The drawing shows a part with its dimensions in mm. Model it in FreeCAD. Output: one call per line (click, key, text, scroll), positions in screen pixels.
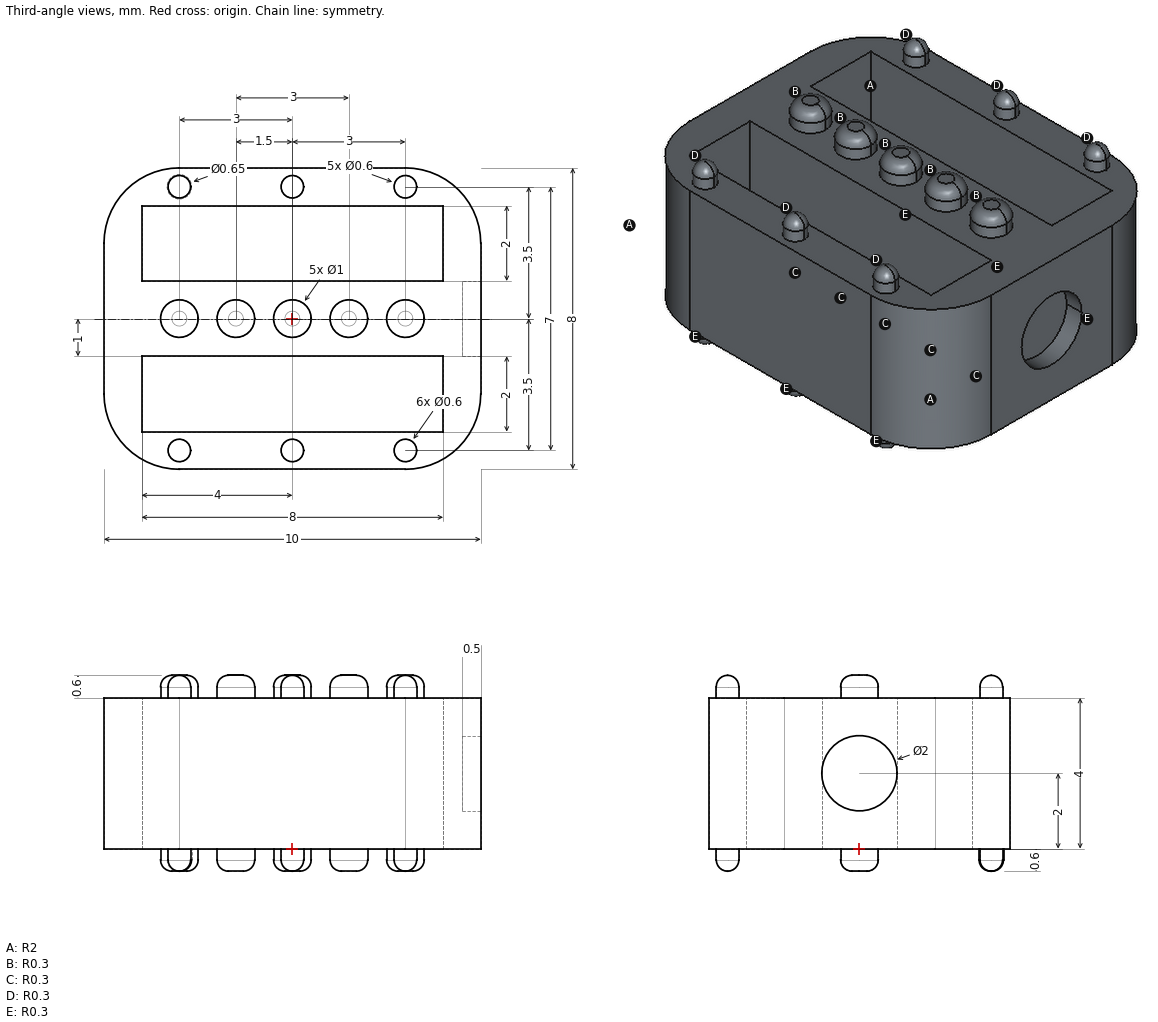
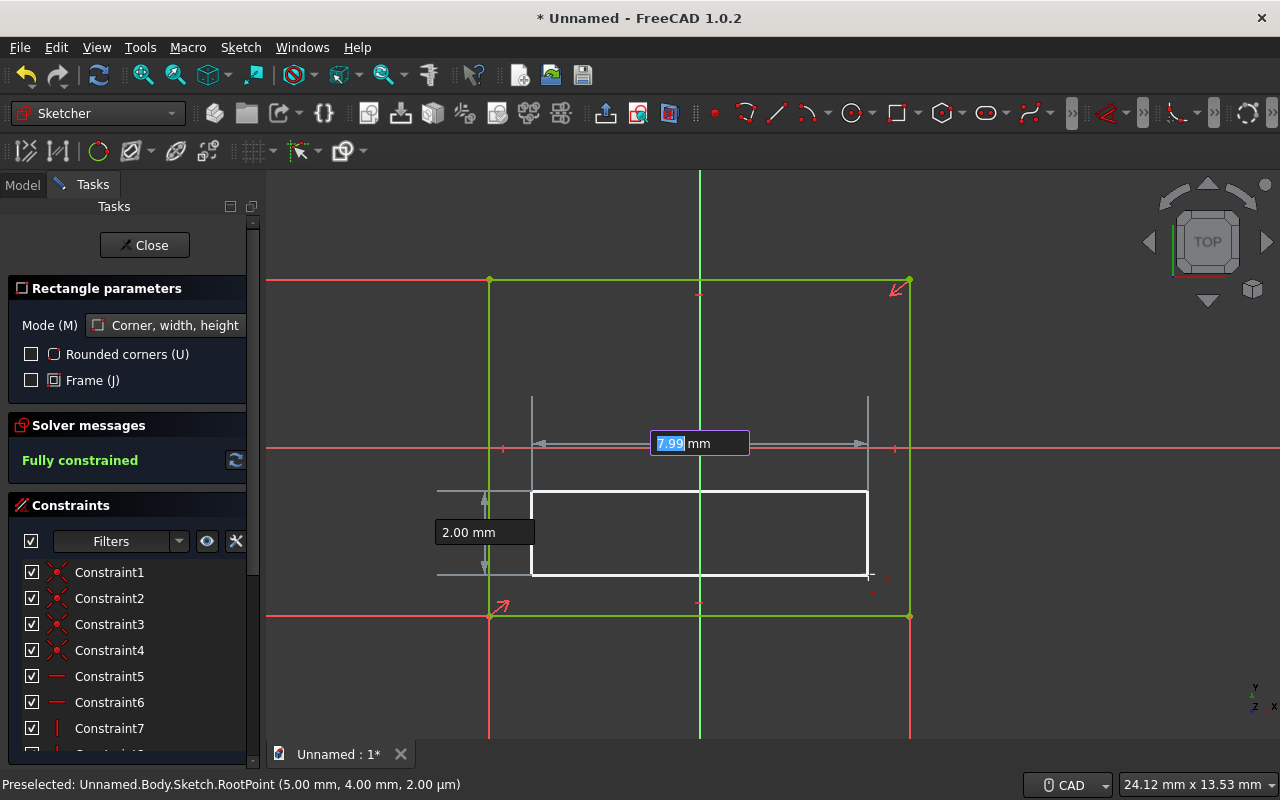
text(8)
key(Tab)
text(2)
key(Return)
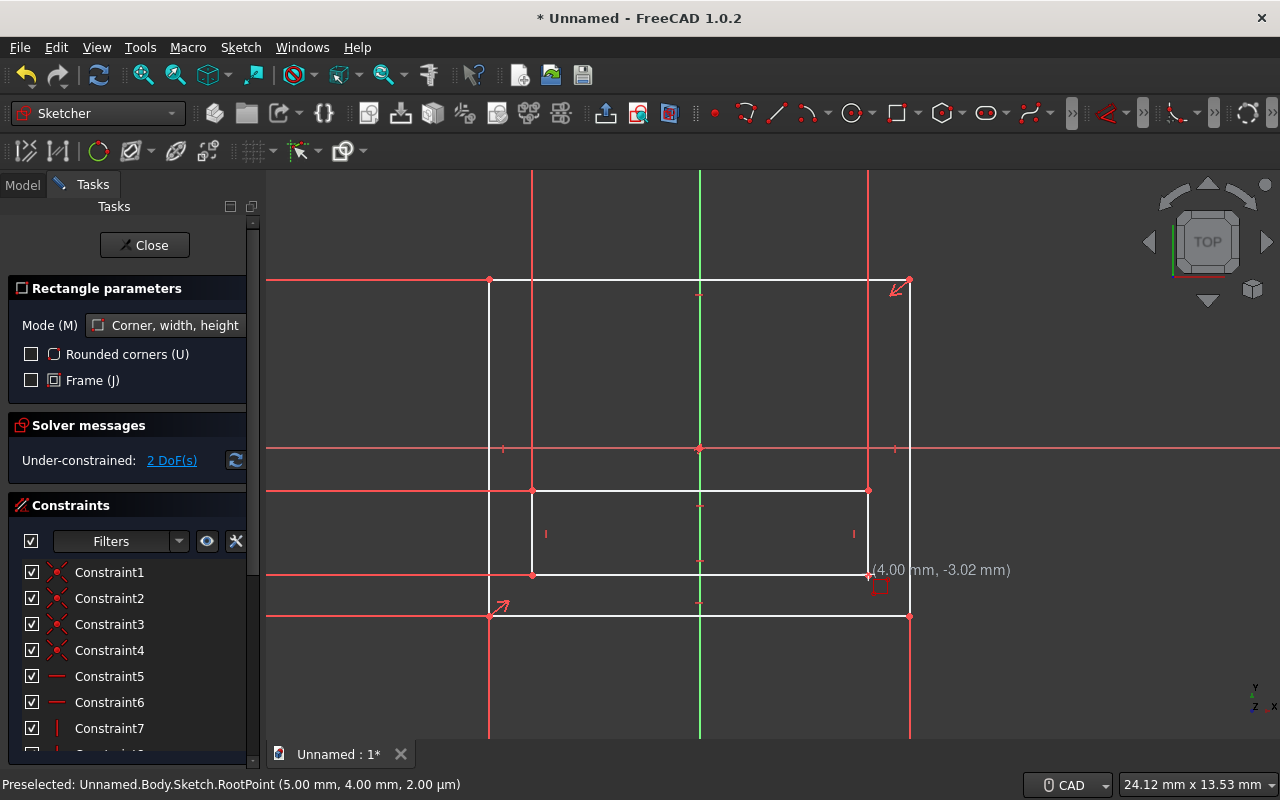
click(532, 322)
move(868, 406)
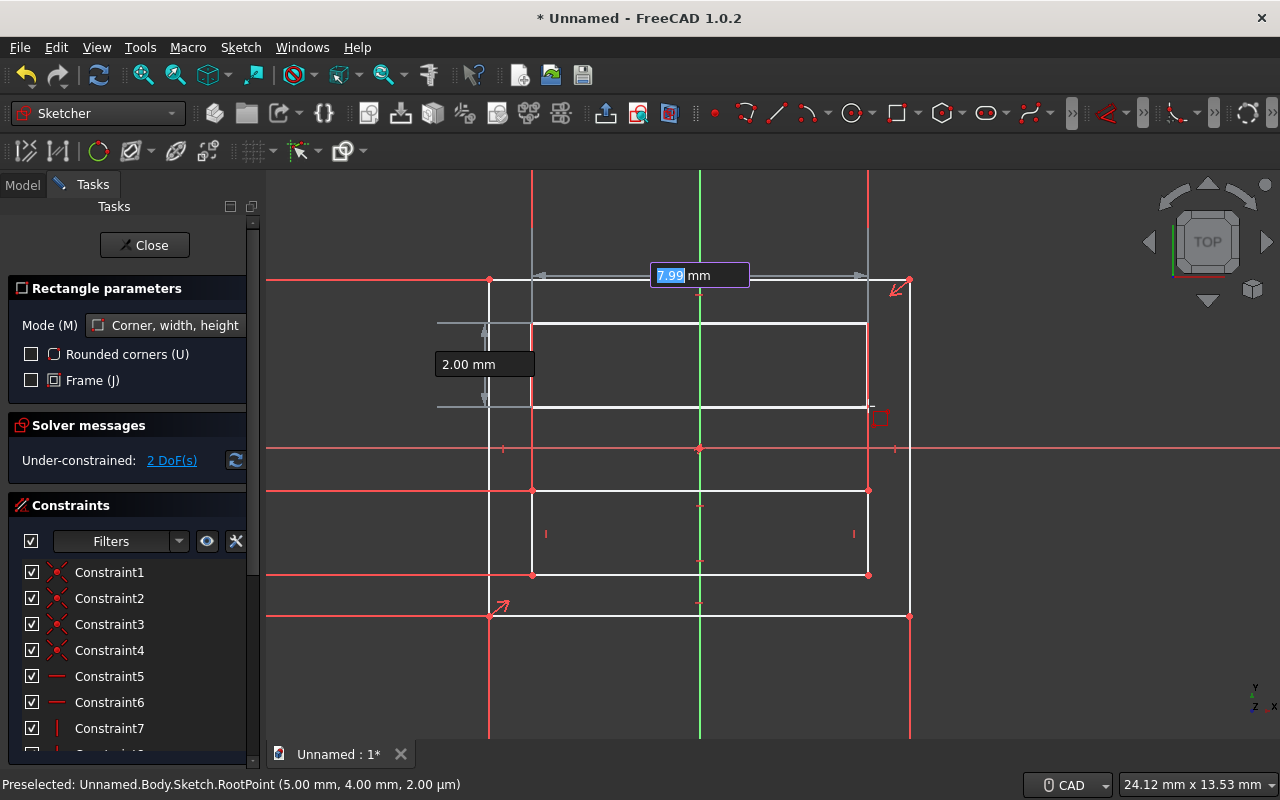
text(8)
key(Tab)
text(2)
key(Return)
key(Escape)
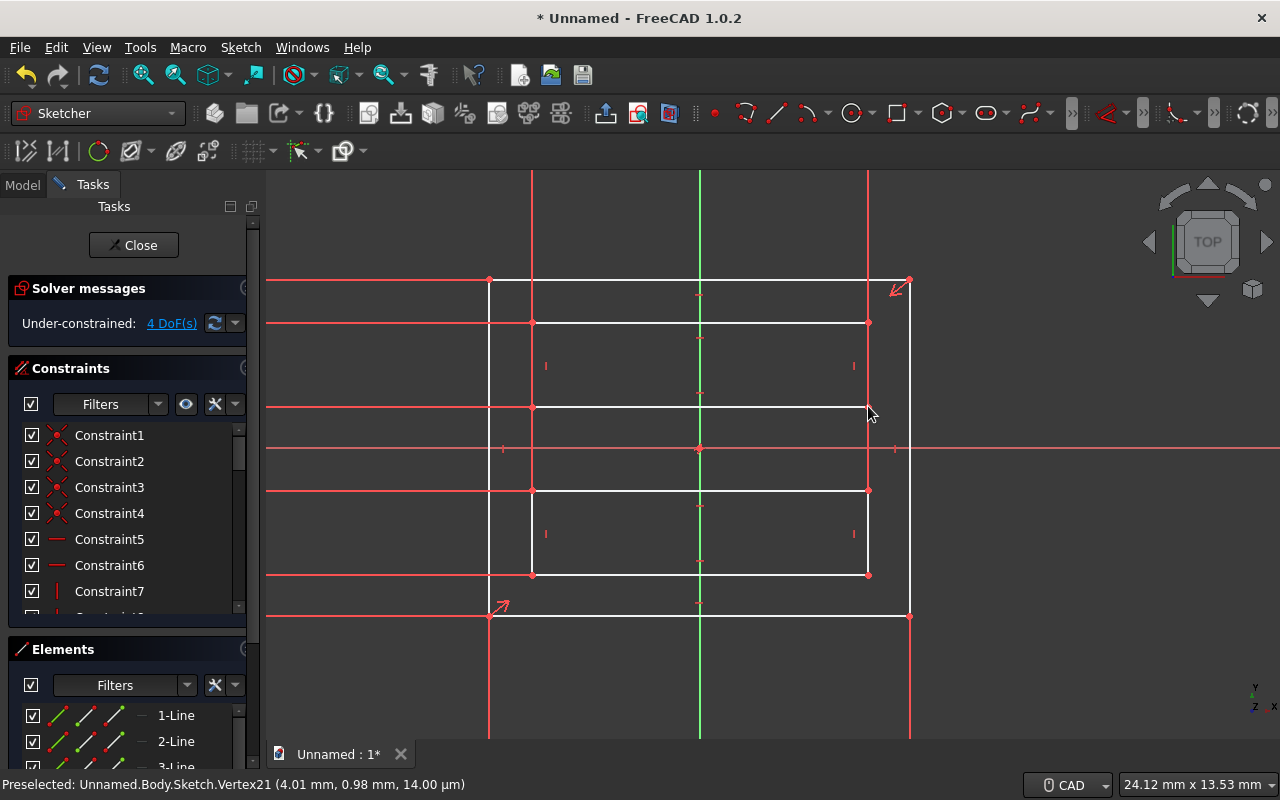
click(532, 575)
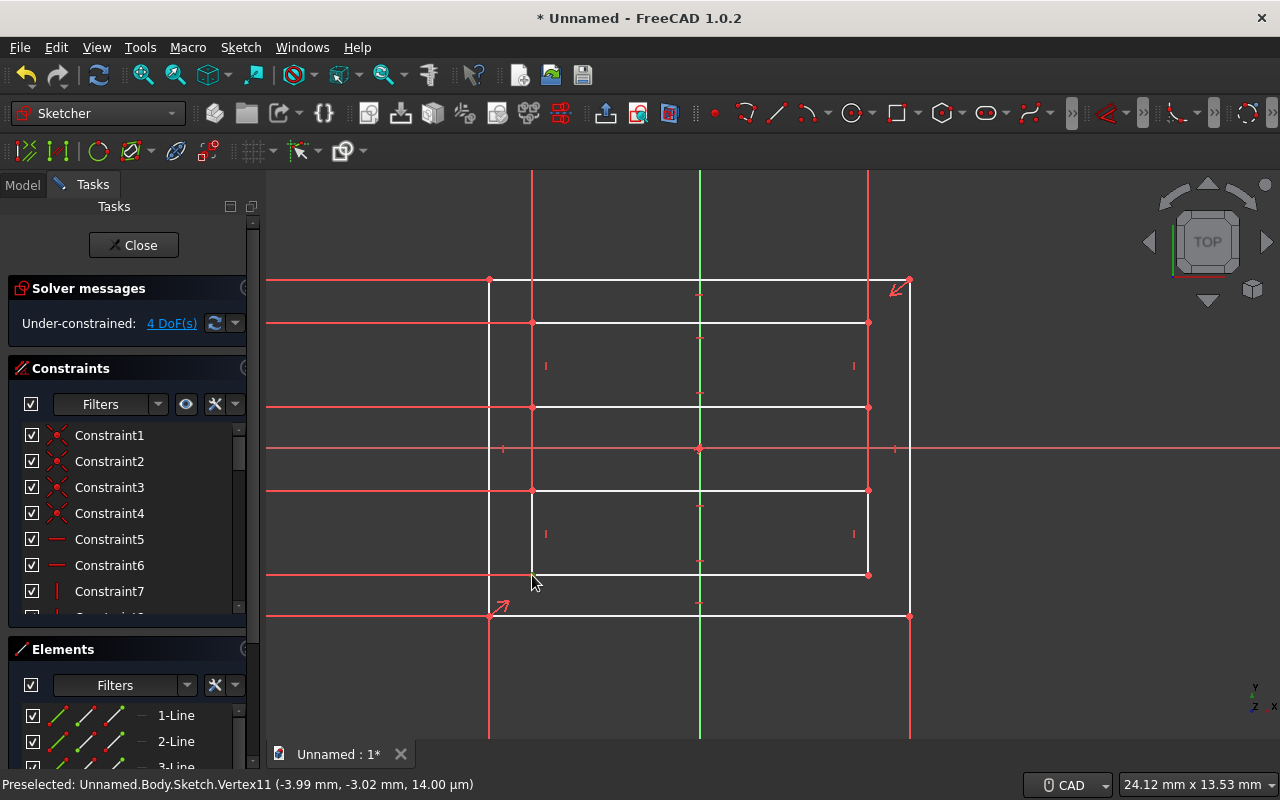
click(532, 323)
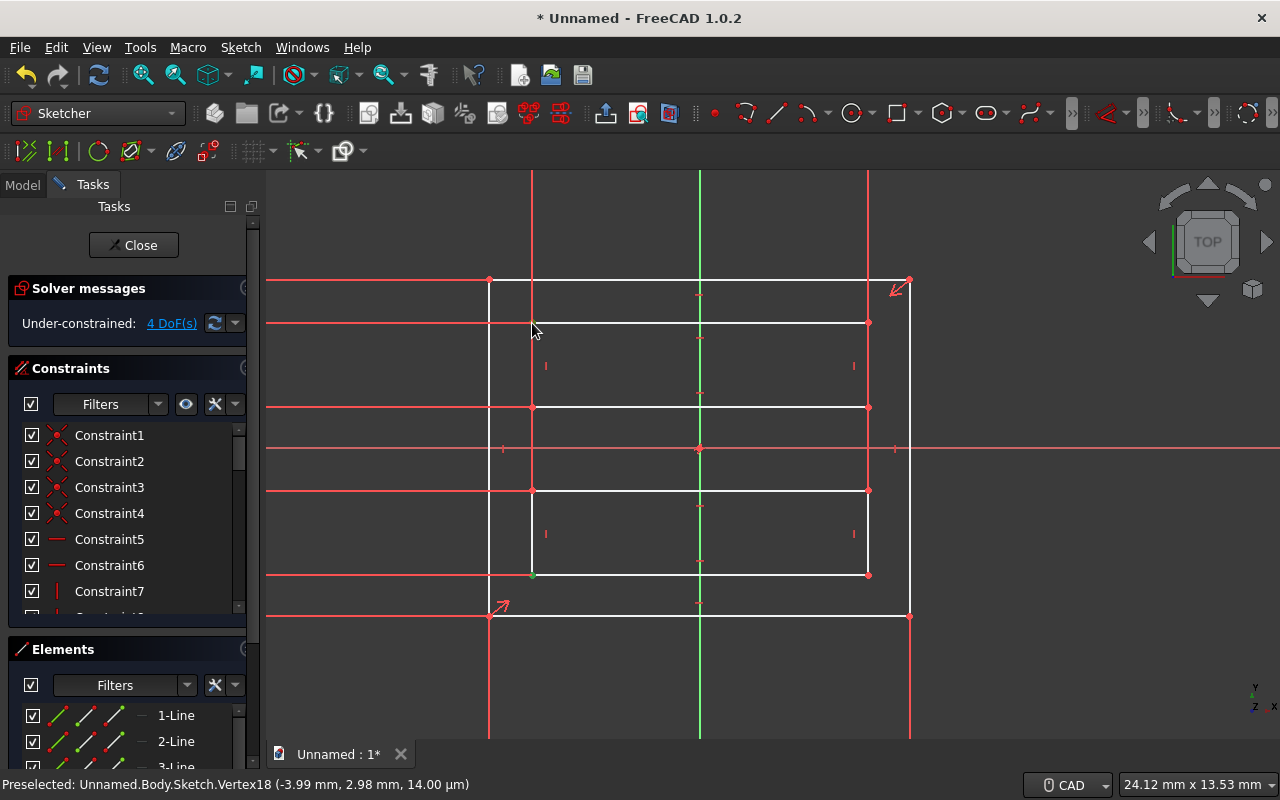
click(353, 448)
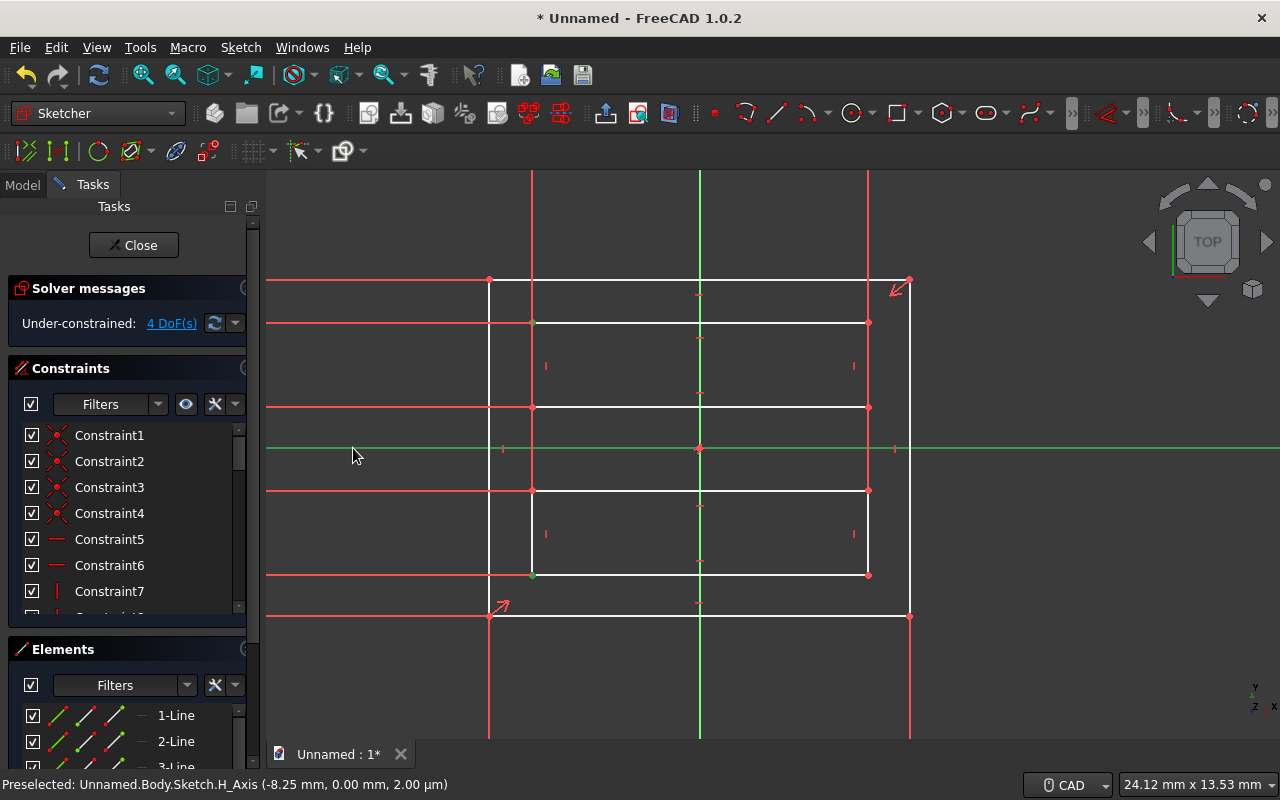
key(s)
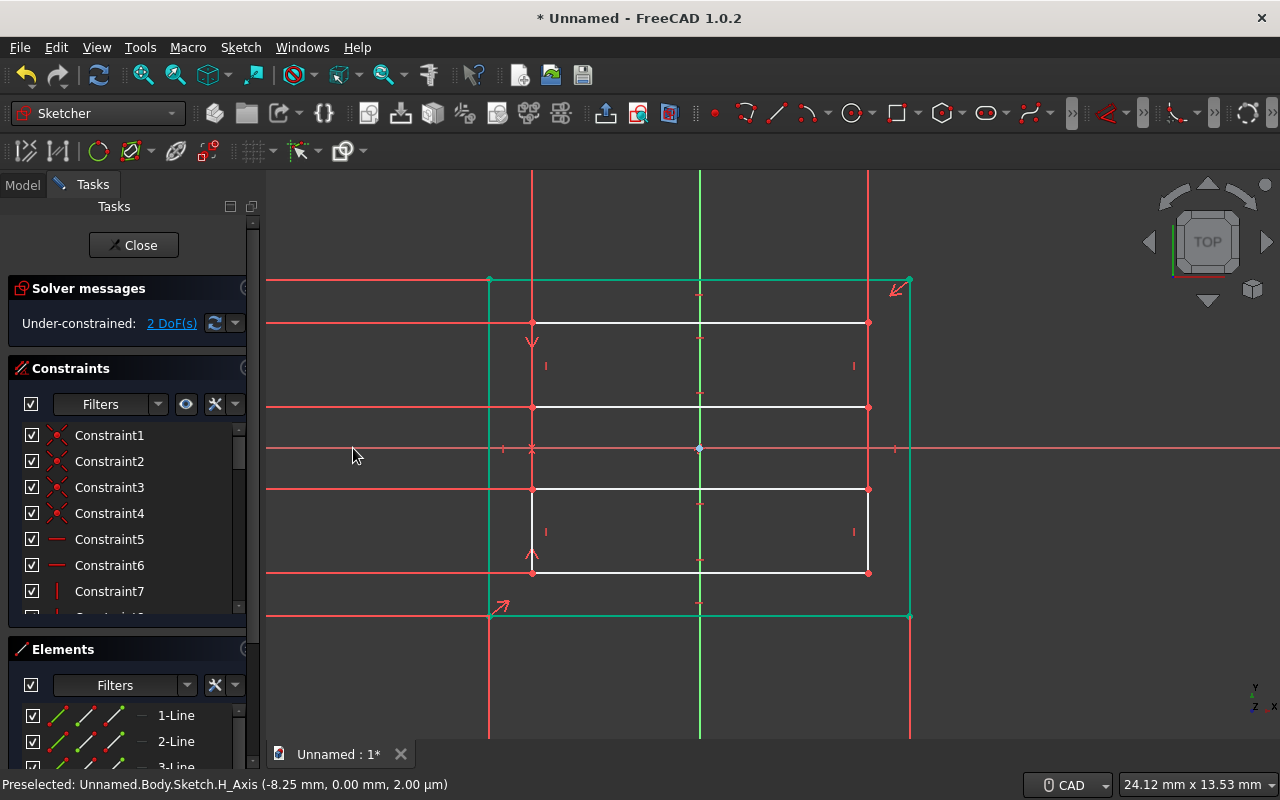
click(532, 489)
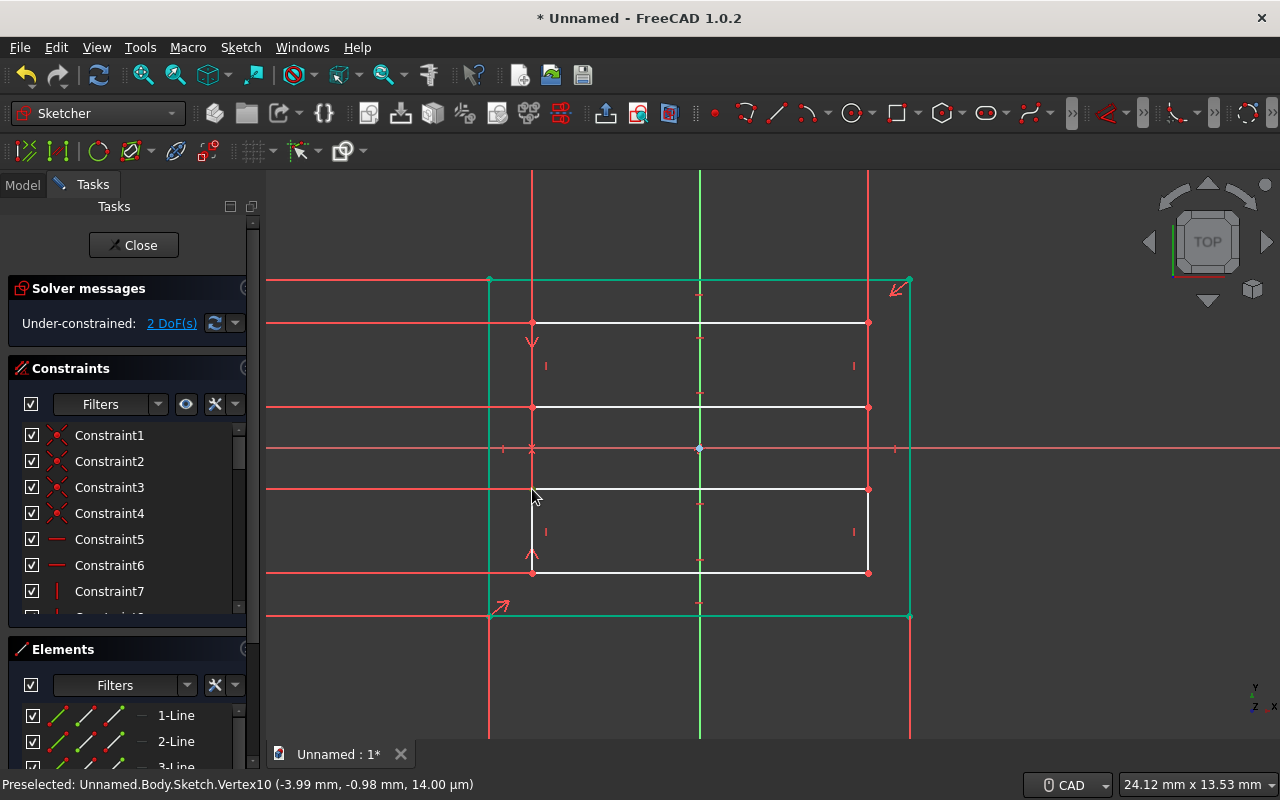
click(1128, 114)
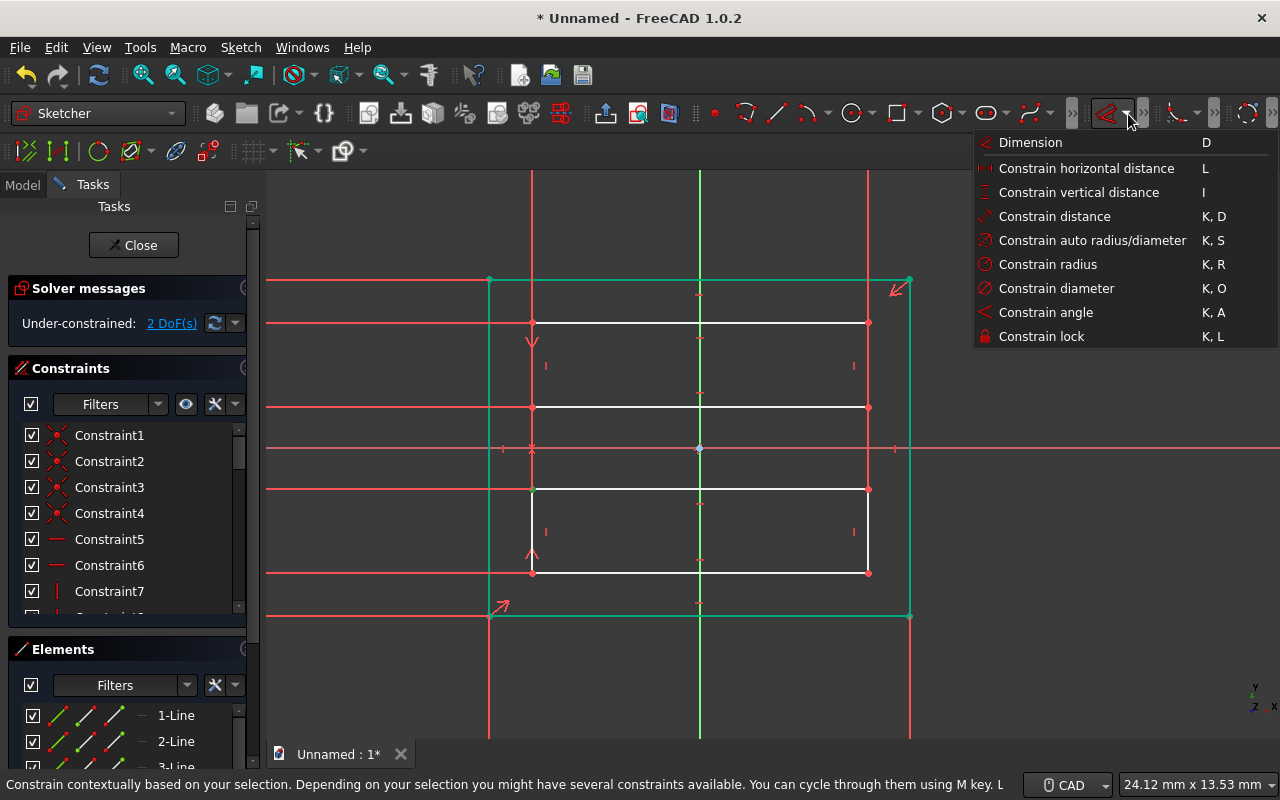
click(1126, 168)